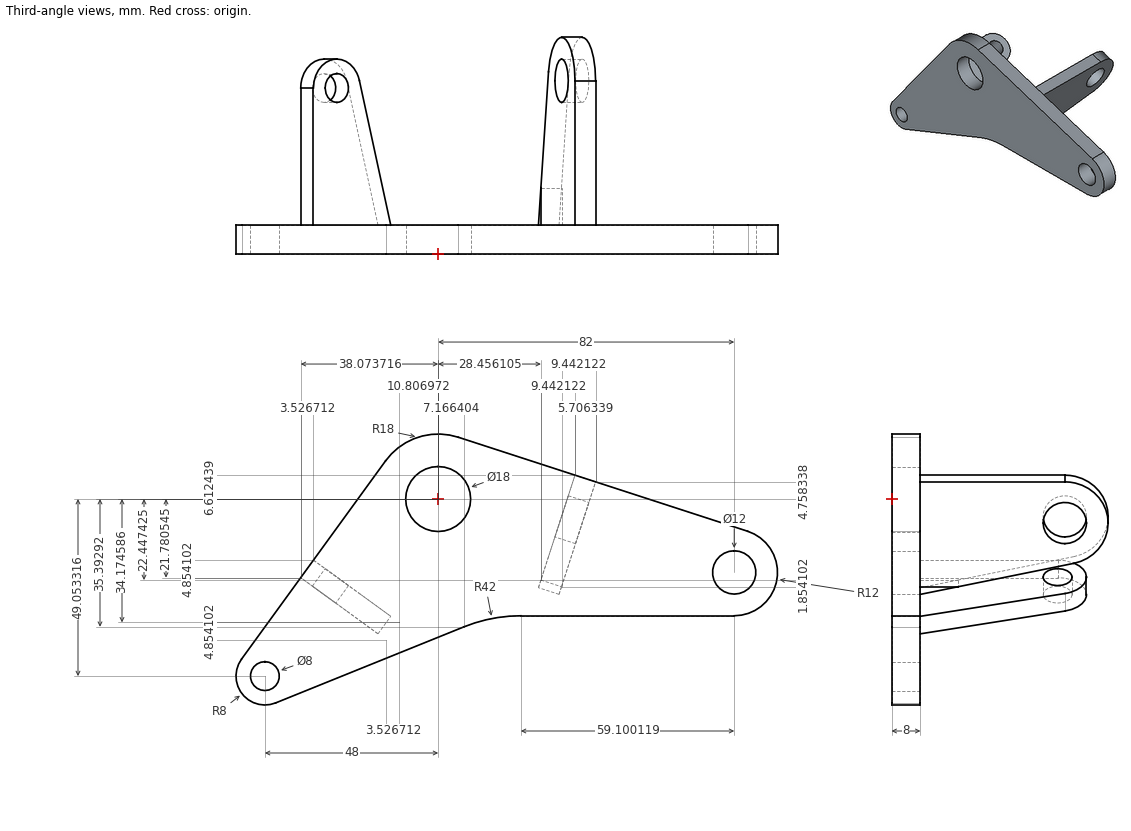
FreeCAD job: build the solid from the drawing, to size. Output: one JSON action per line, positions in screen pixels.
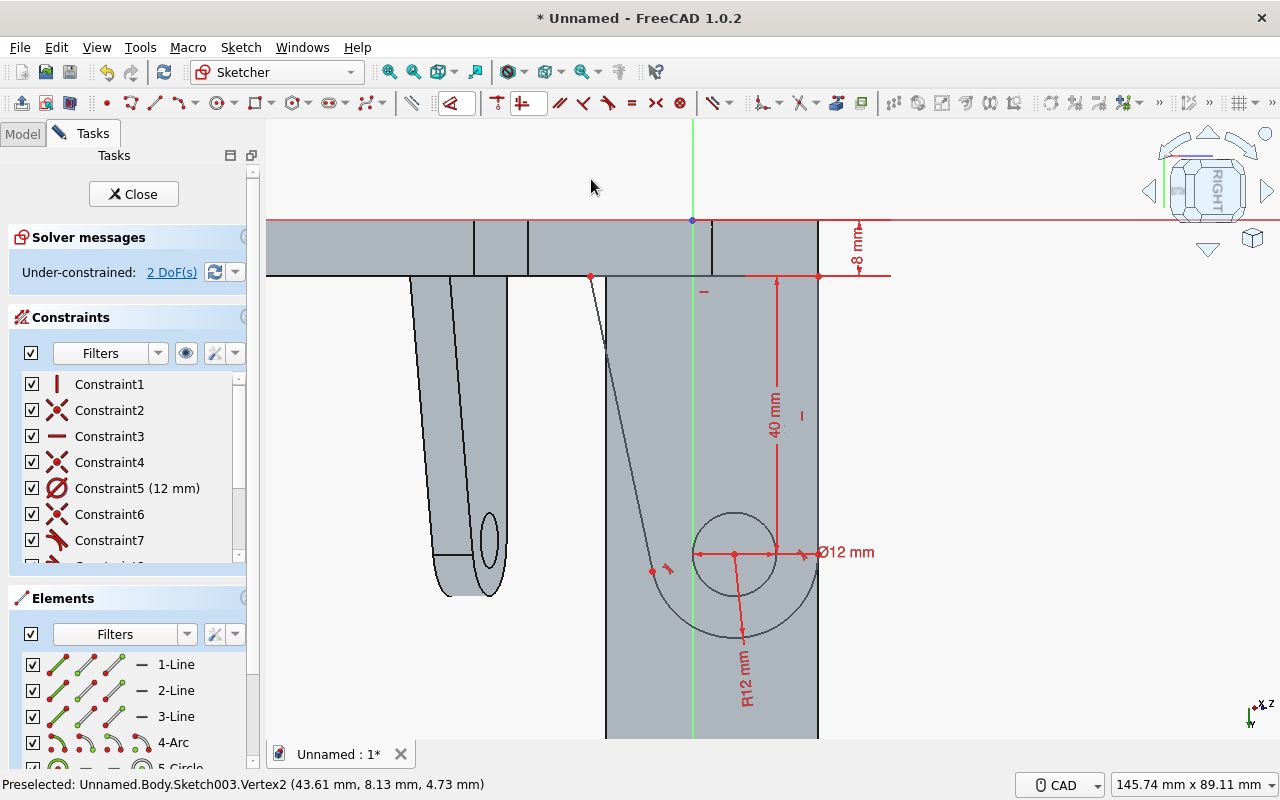
{"action": "left_click", "coordinate": [750, 276]}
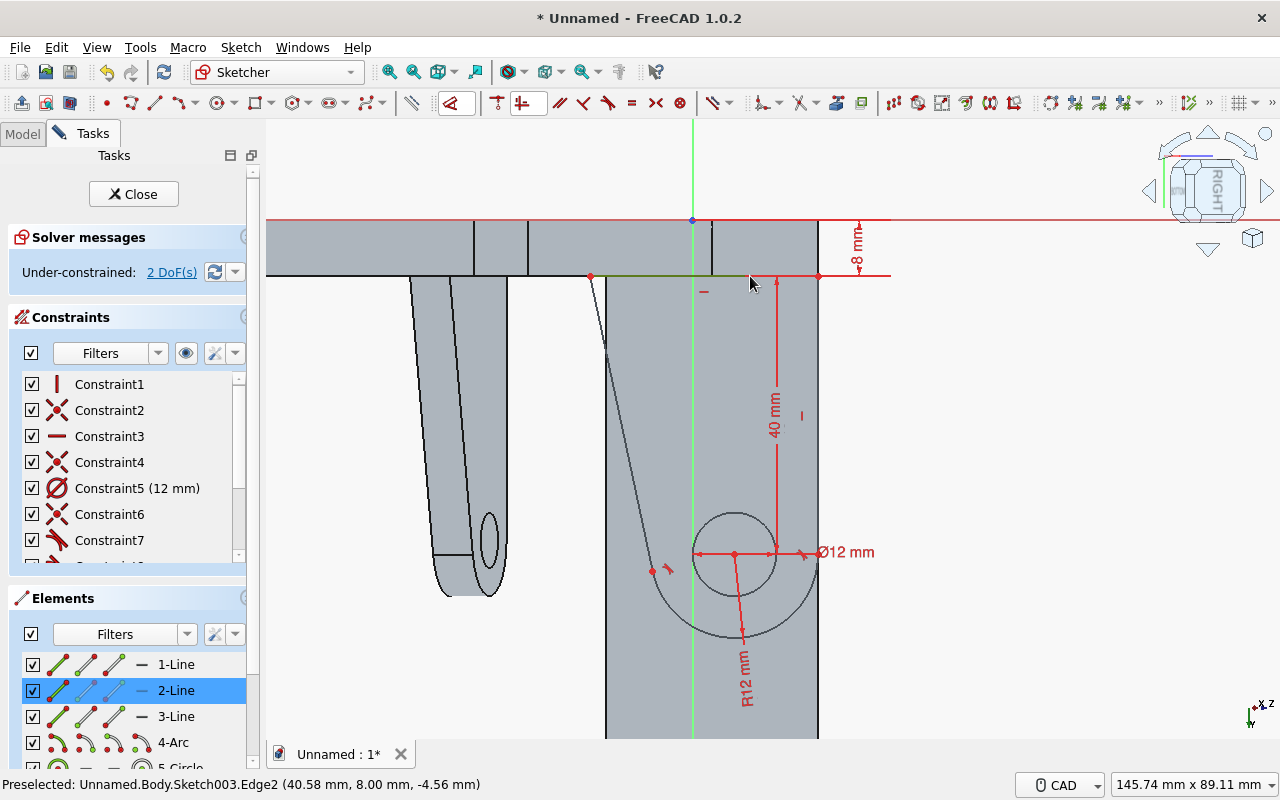
{"action": "left_click", "coordinate": [470, 104]}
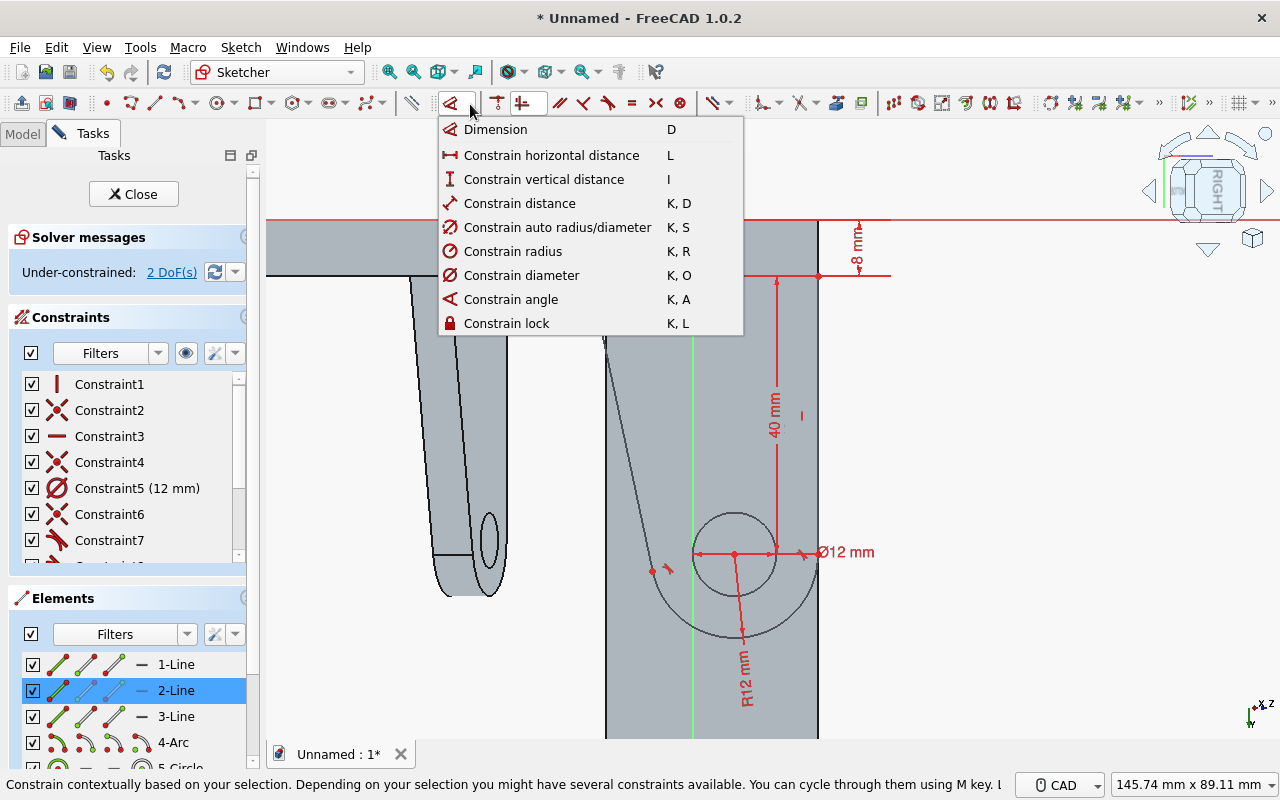
{"action": "left_click", "coordinate": [591, 155]}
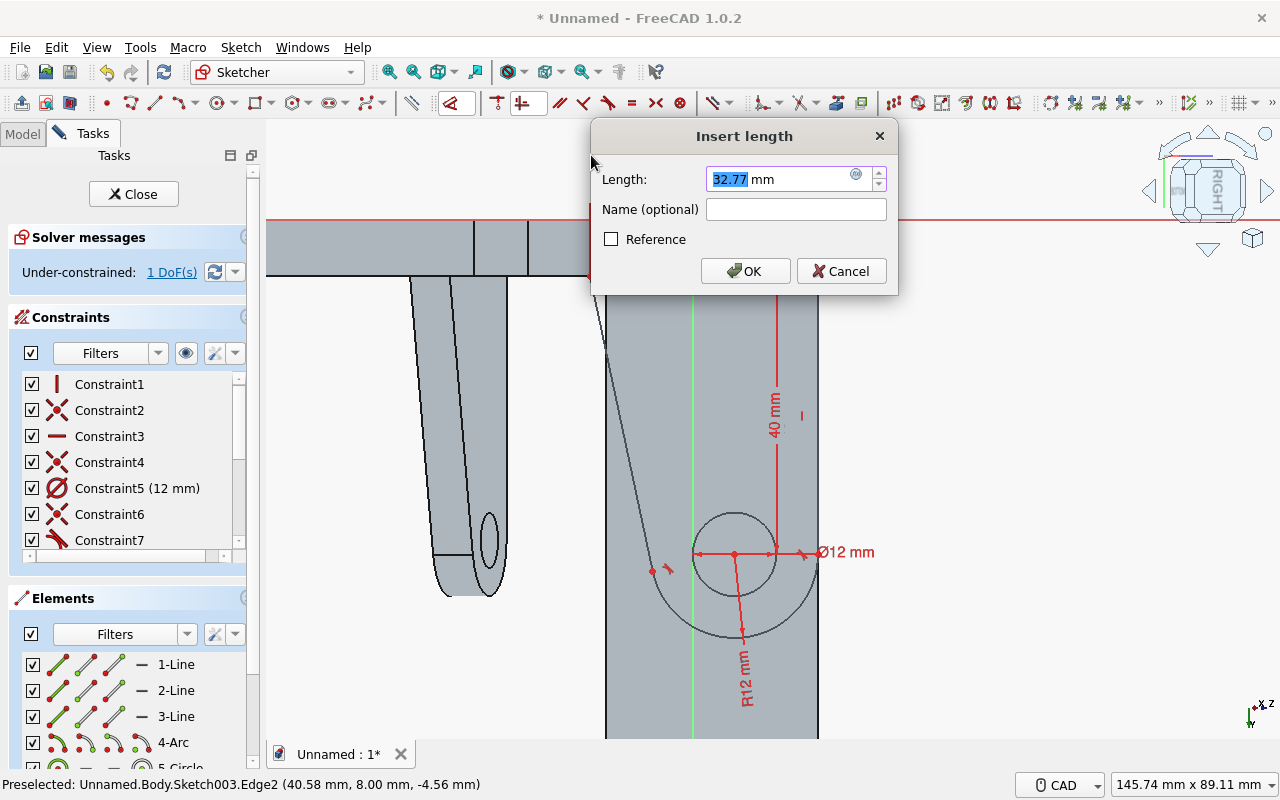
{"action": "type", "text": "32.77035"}
{"action": "key", "text": "Return"}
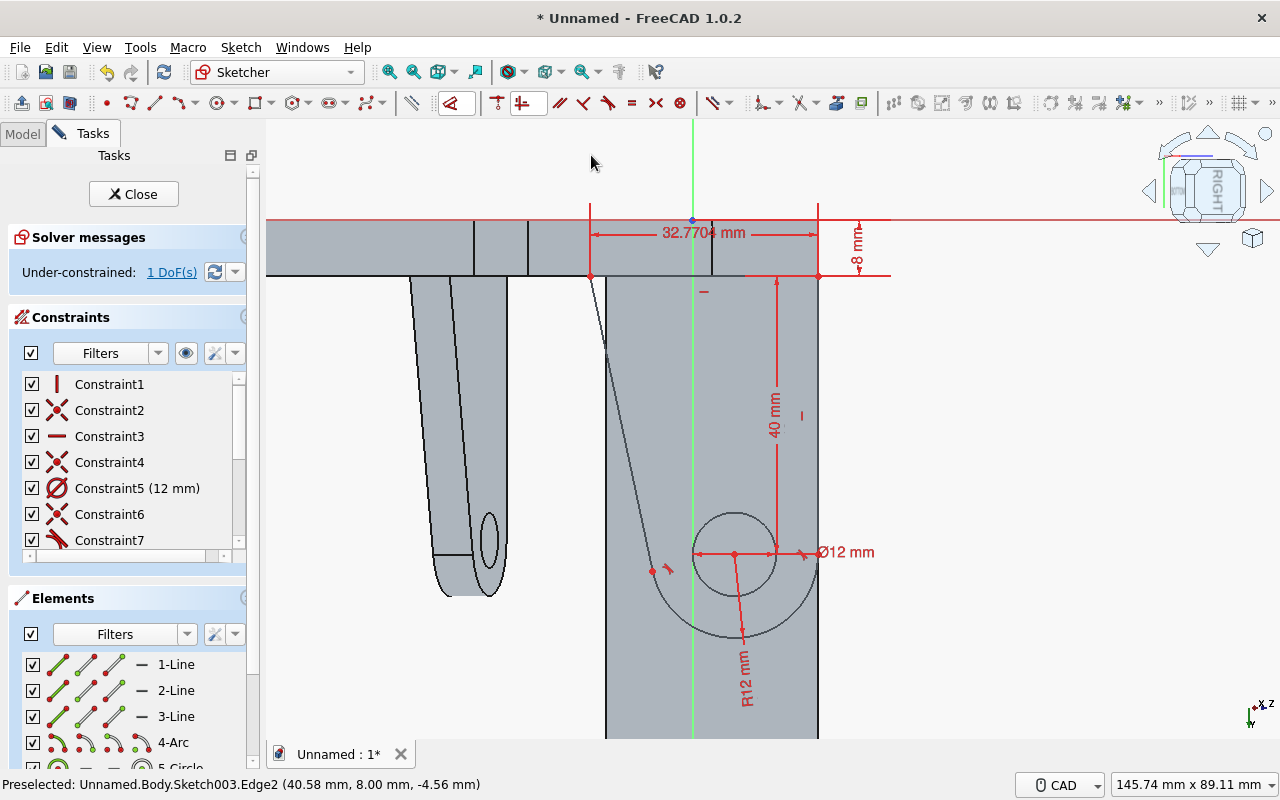
{"action": "left_click", "coordinate": [735, 554]}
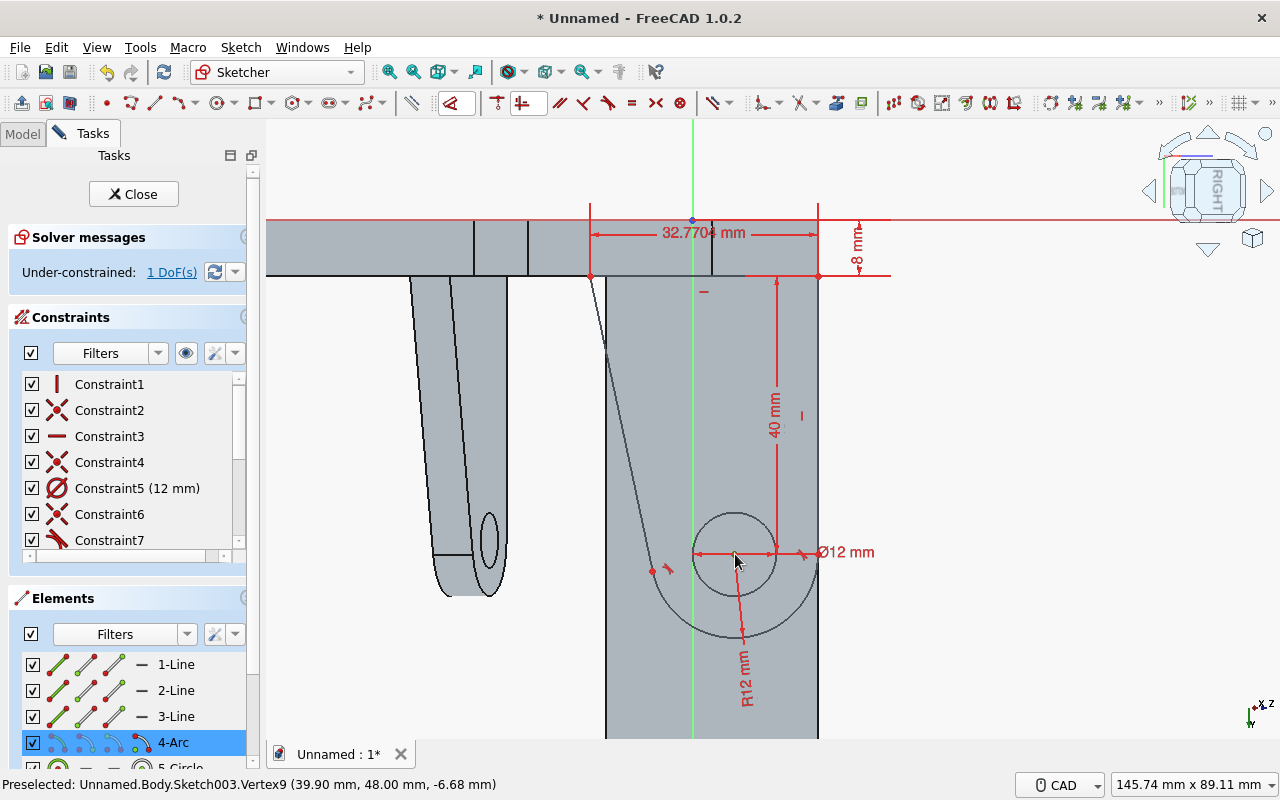
{"action": "left_click", "coordinate": [470, 104]}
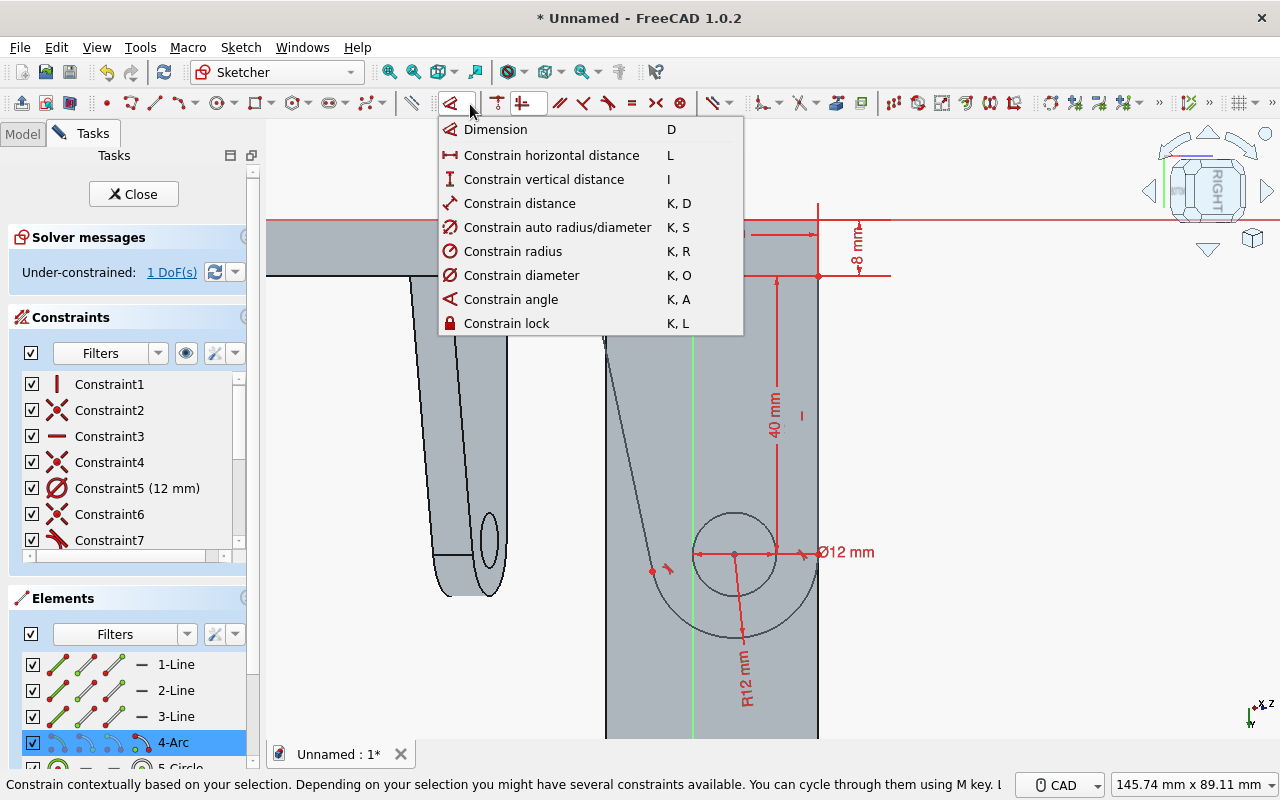
{"action": "left_click", "coordinate": [591, 155]}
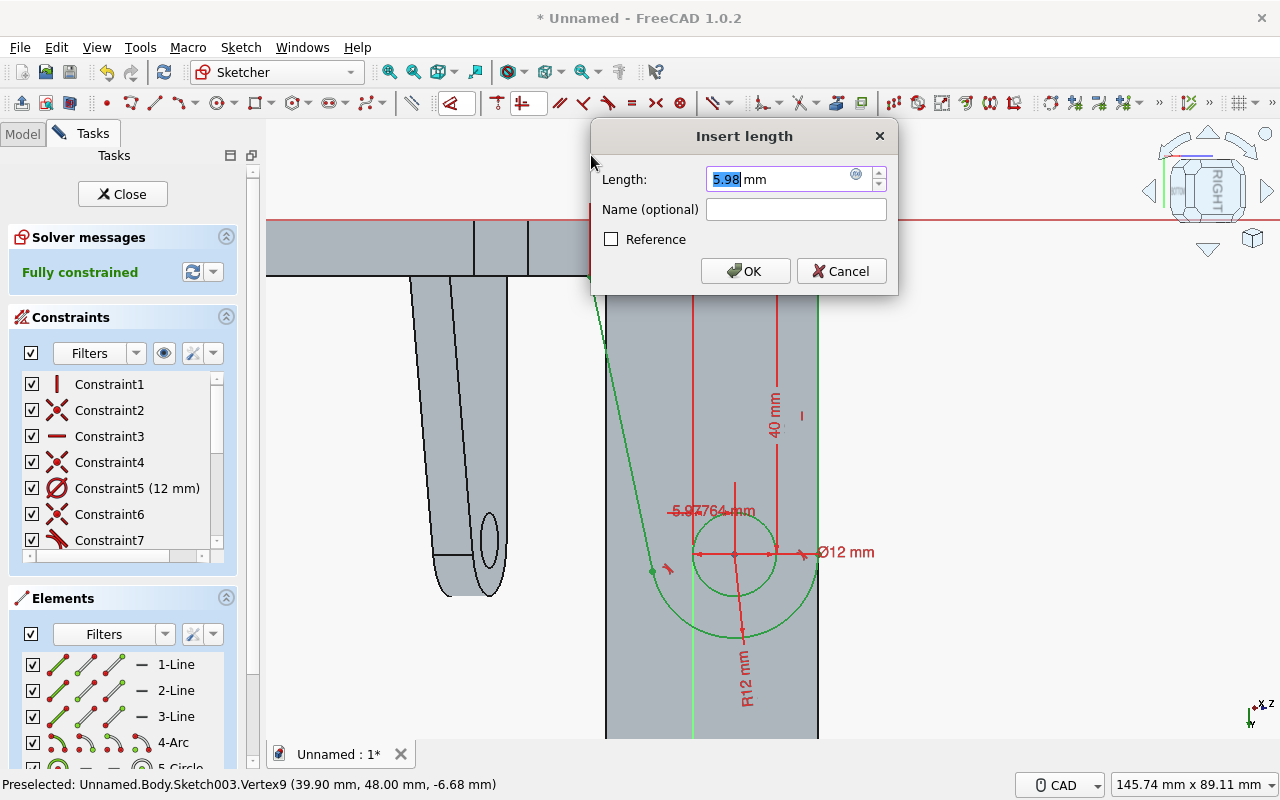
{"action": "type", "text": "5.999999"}
{"action": "key", "text": "Return"}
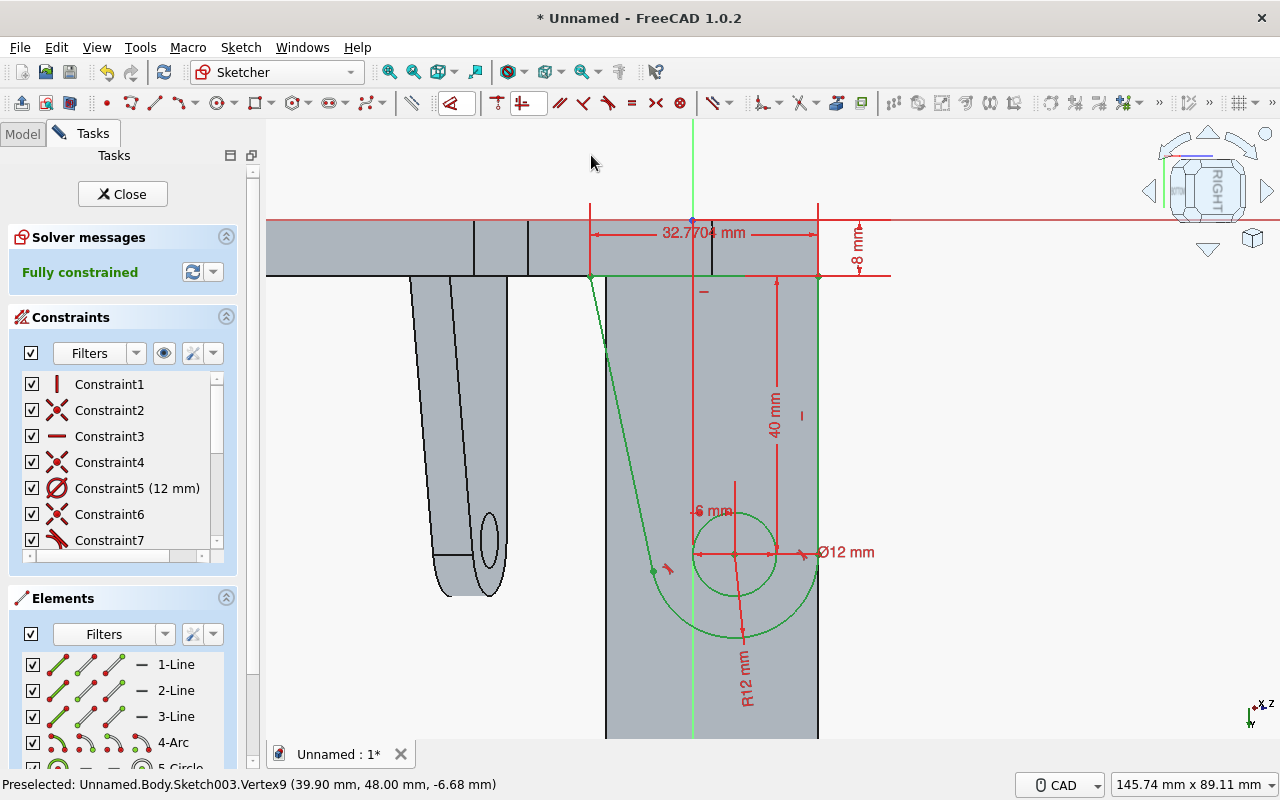
{"action": "left_click", "coordinate": [123, 194]}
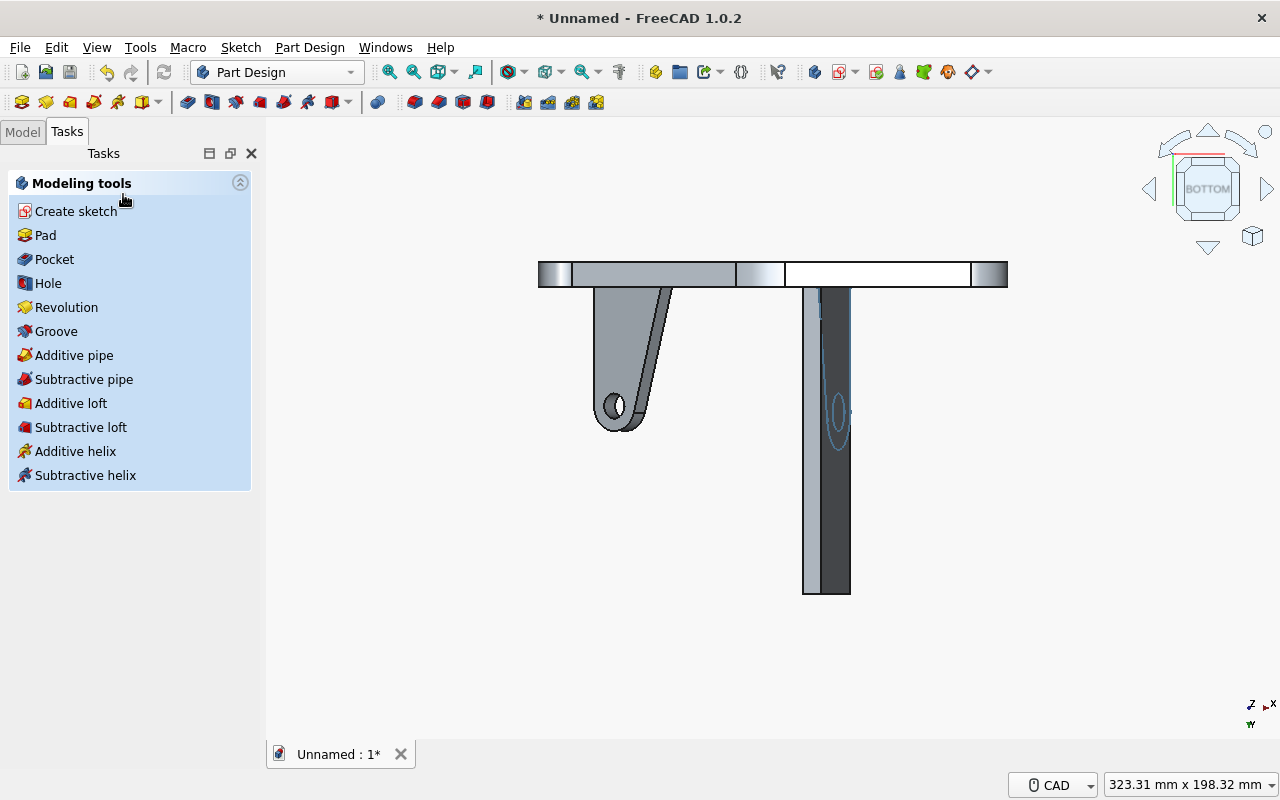
{"action": "left_click", "coordinate": [22, 102]}